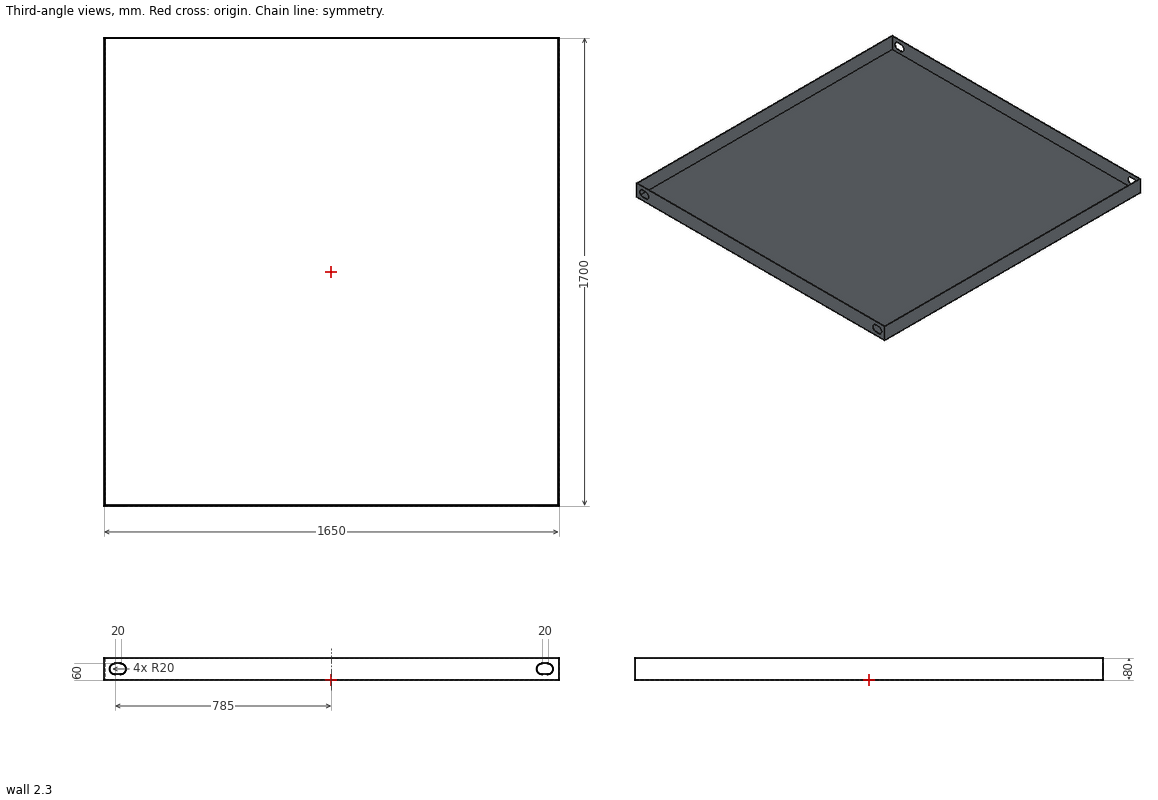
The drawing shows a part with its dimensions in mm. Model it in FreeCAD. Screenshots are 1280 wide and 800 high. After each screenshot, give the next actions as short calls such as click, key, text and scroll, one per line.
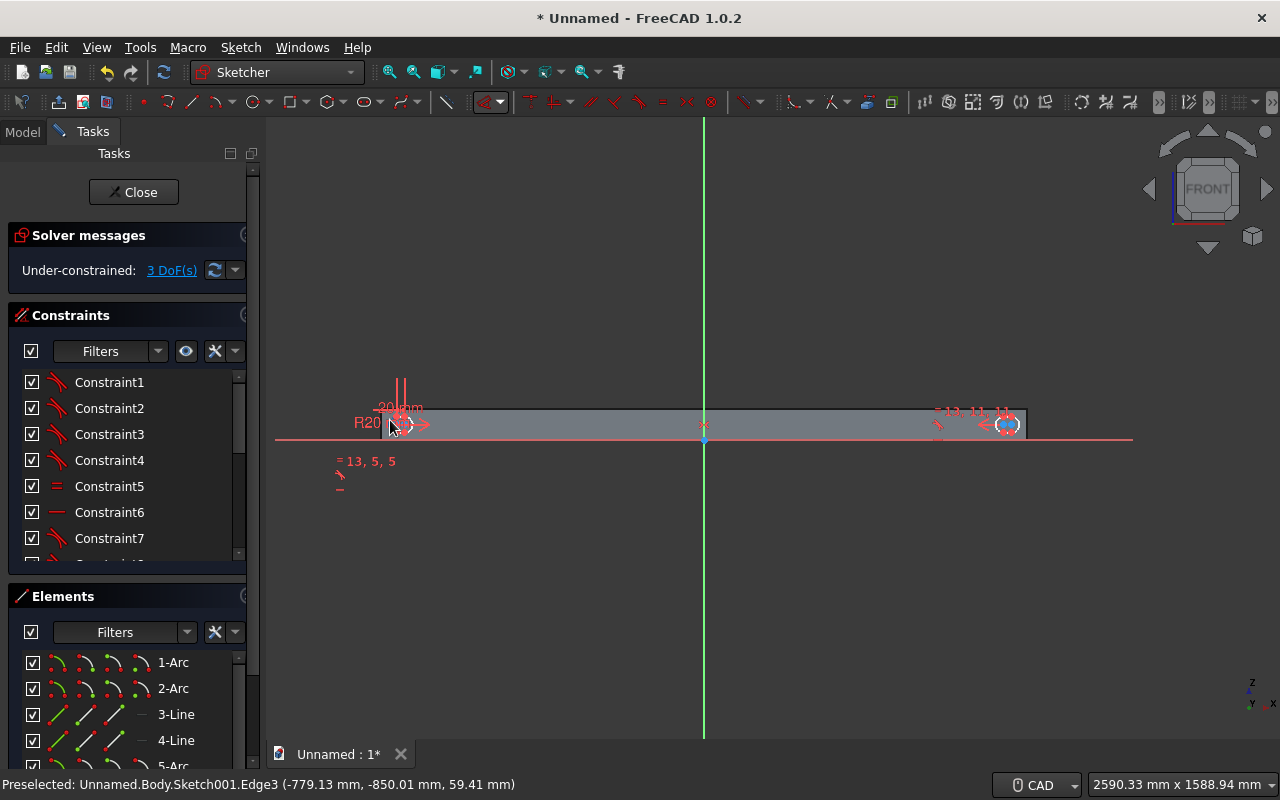
scroll(1006, 417, up, 9)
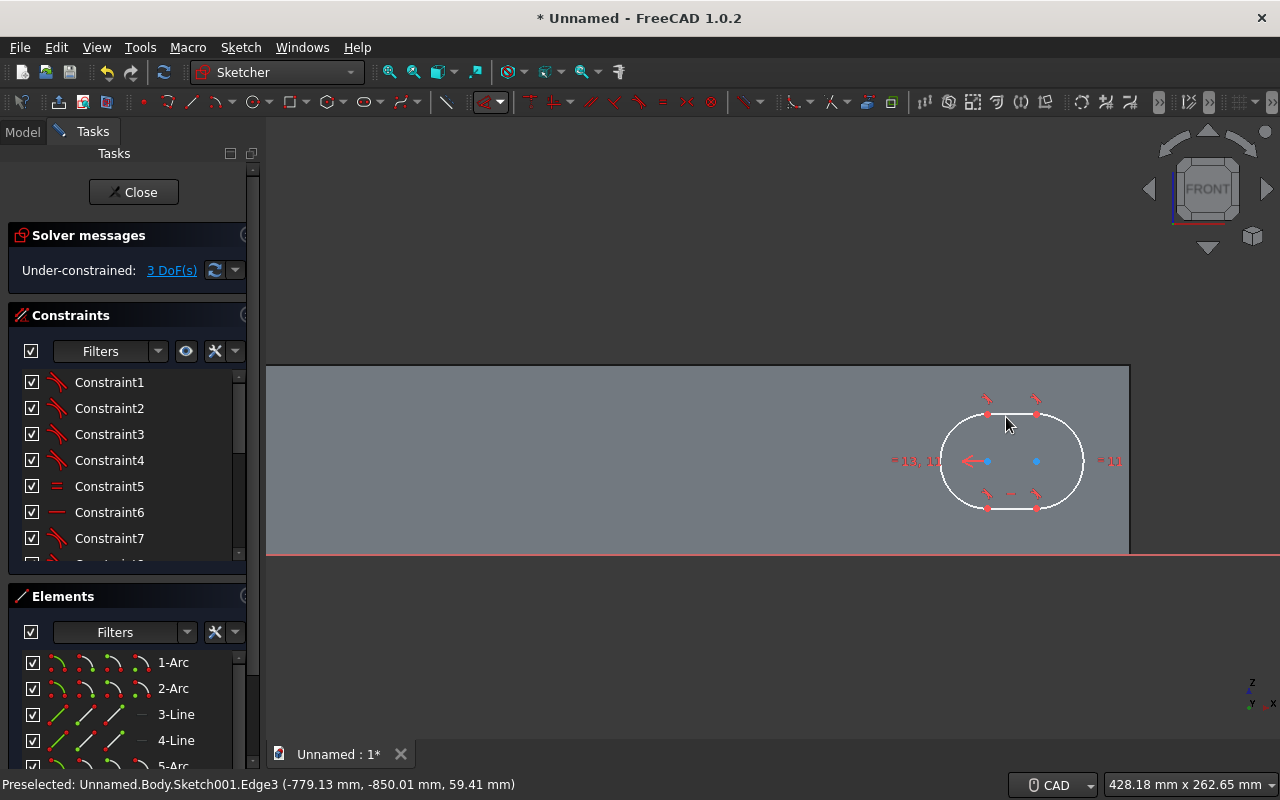
click(1002, 414)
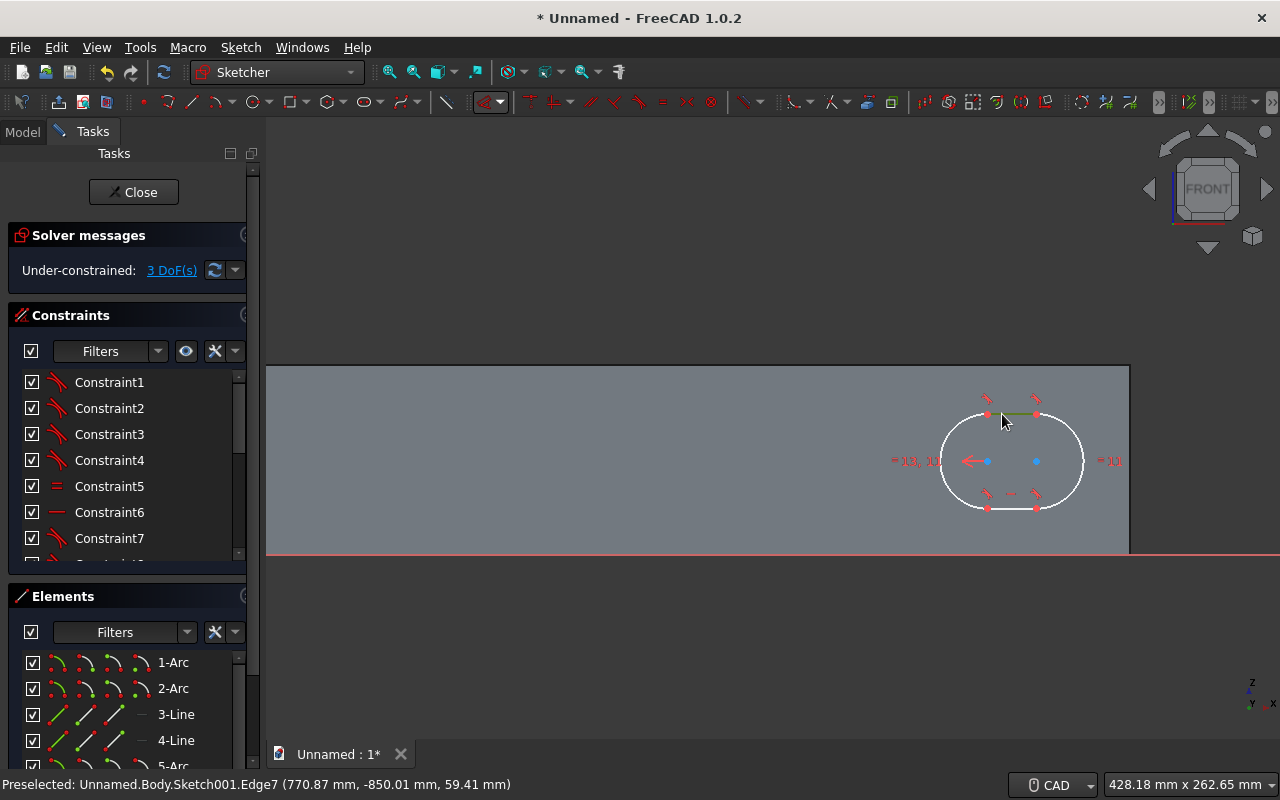
key(l)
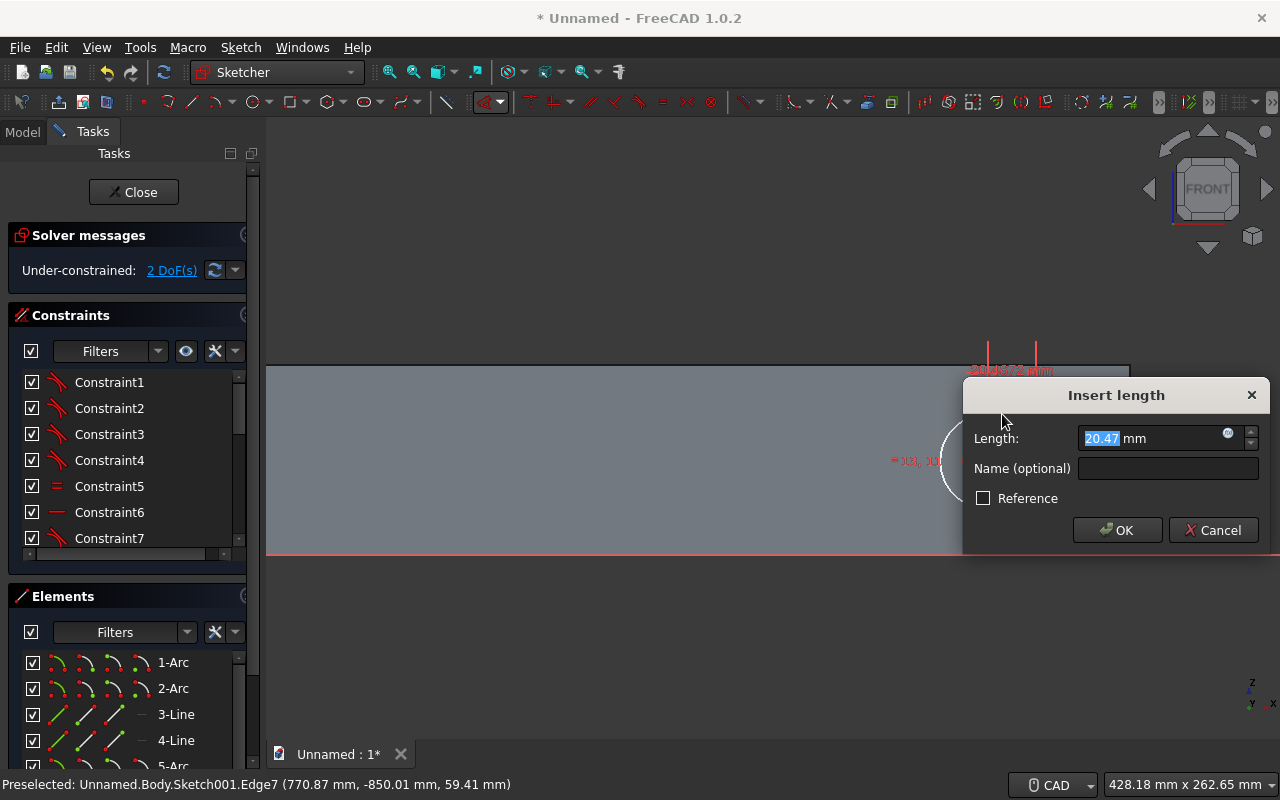
text(20)
key(Return)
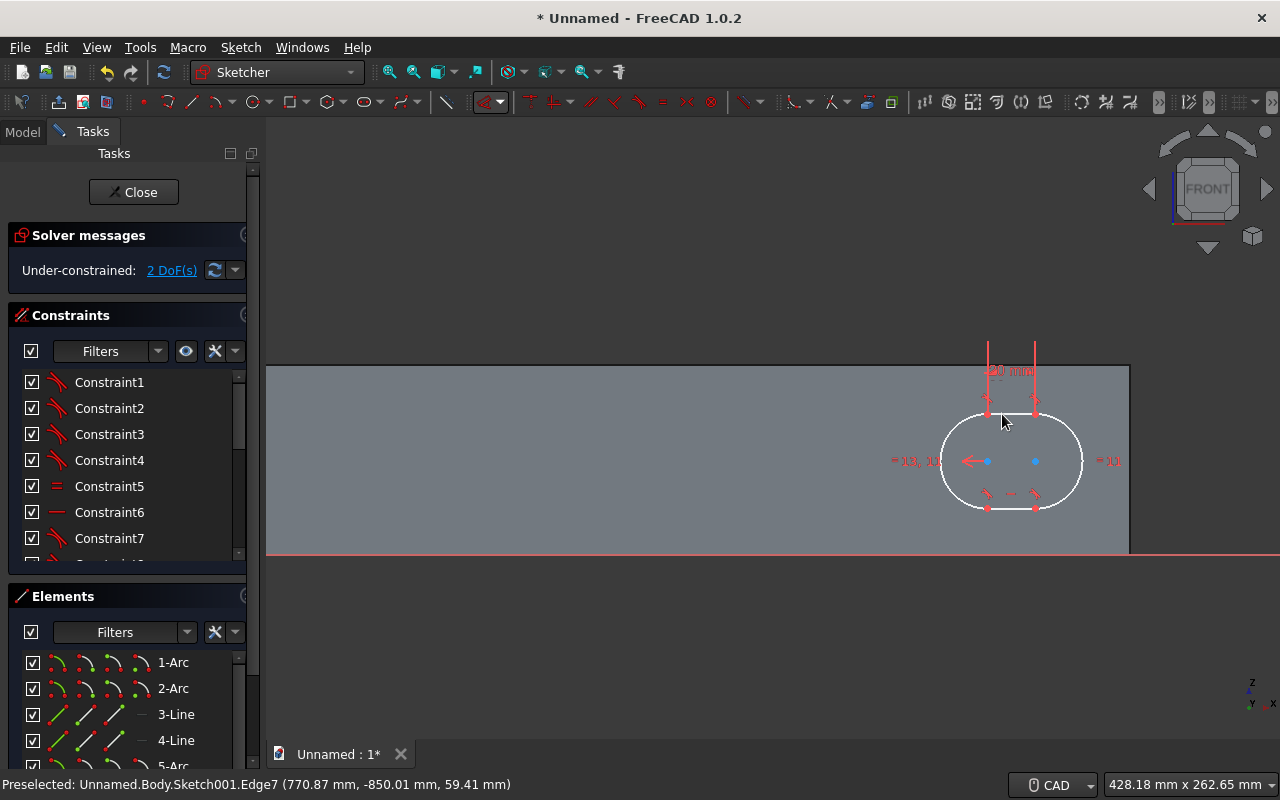
scroll(1007, 417, down, 9)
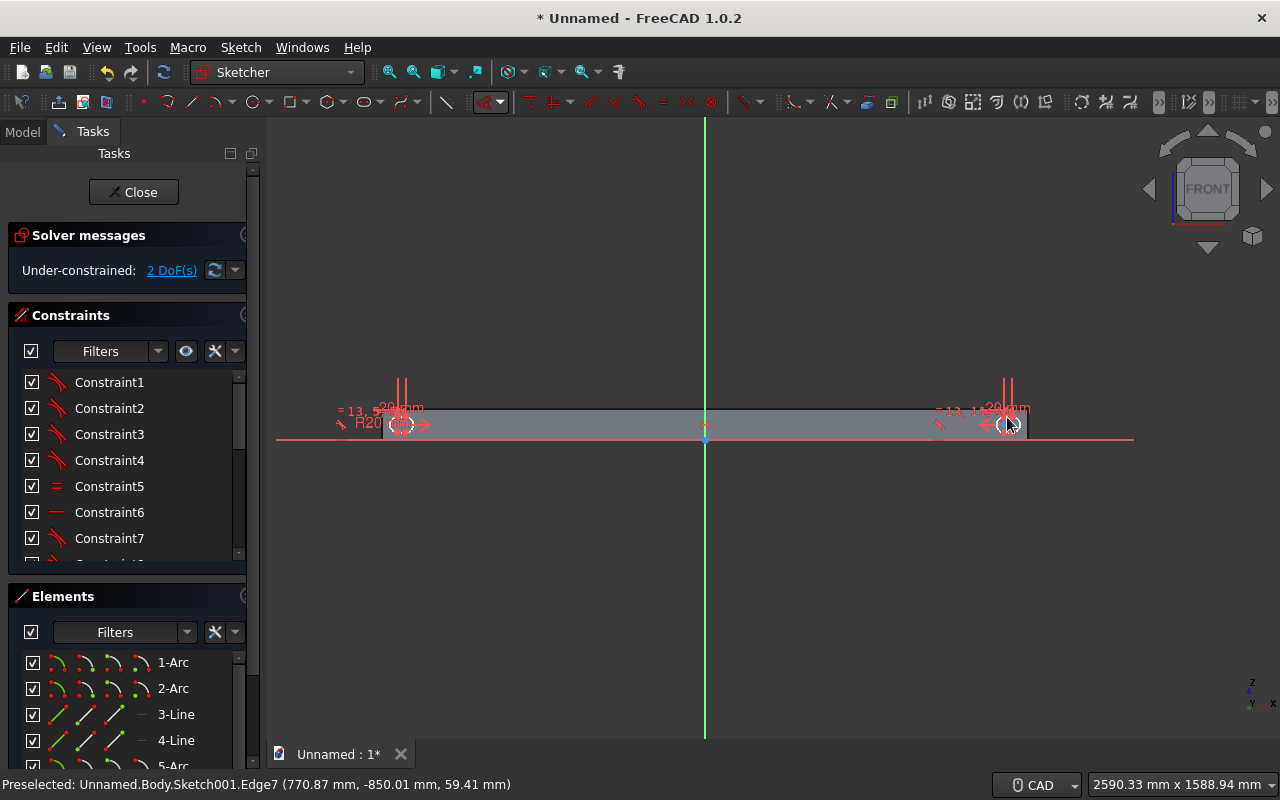
scroll(398, 417, up, 3)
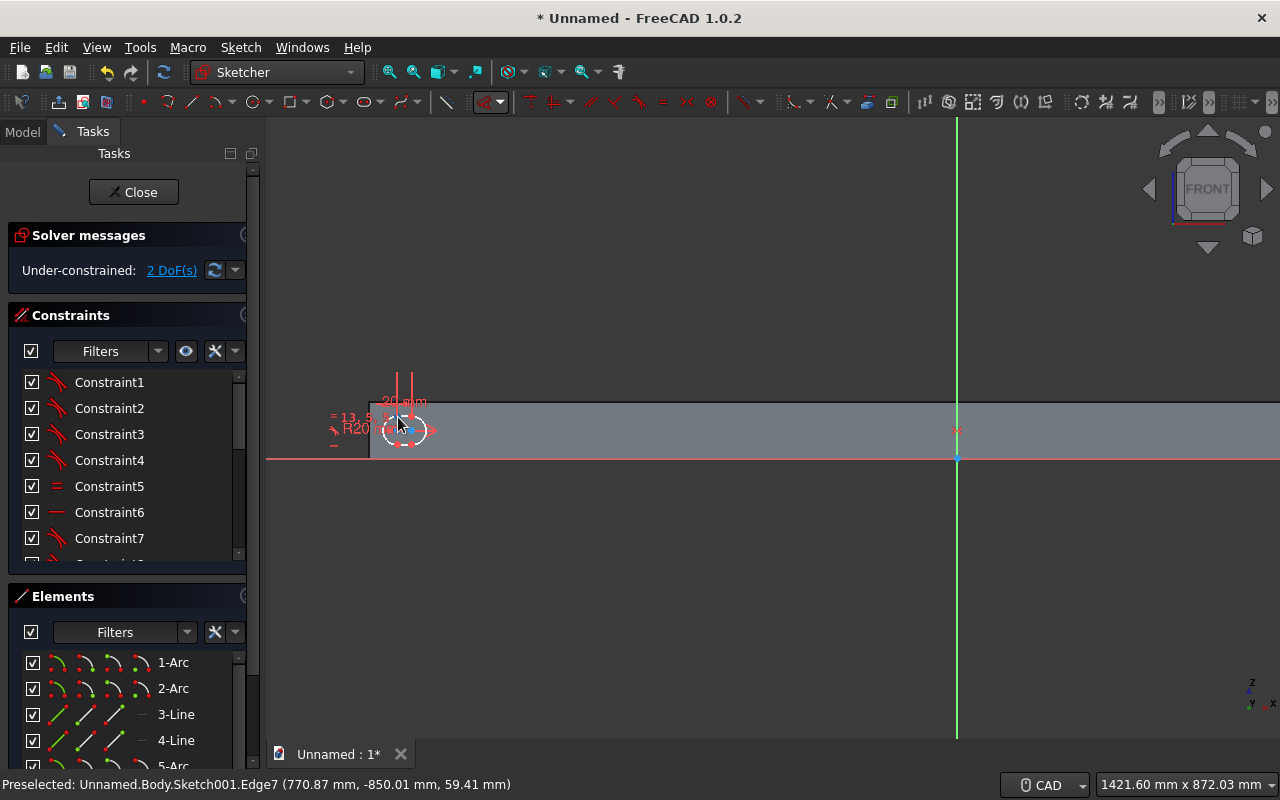
click(397, 416)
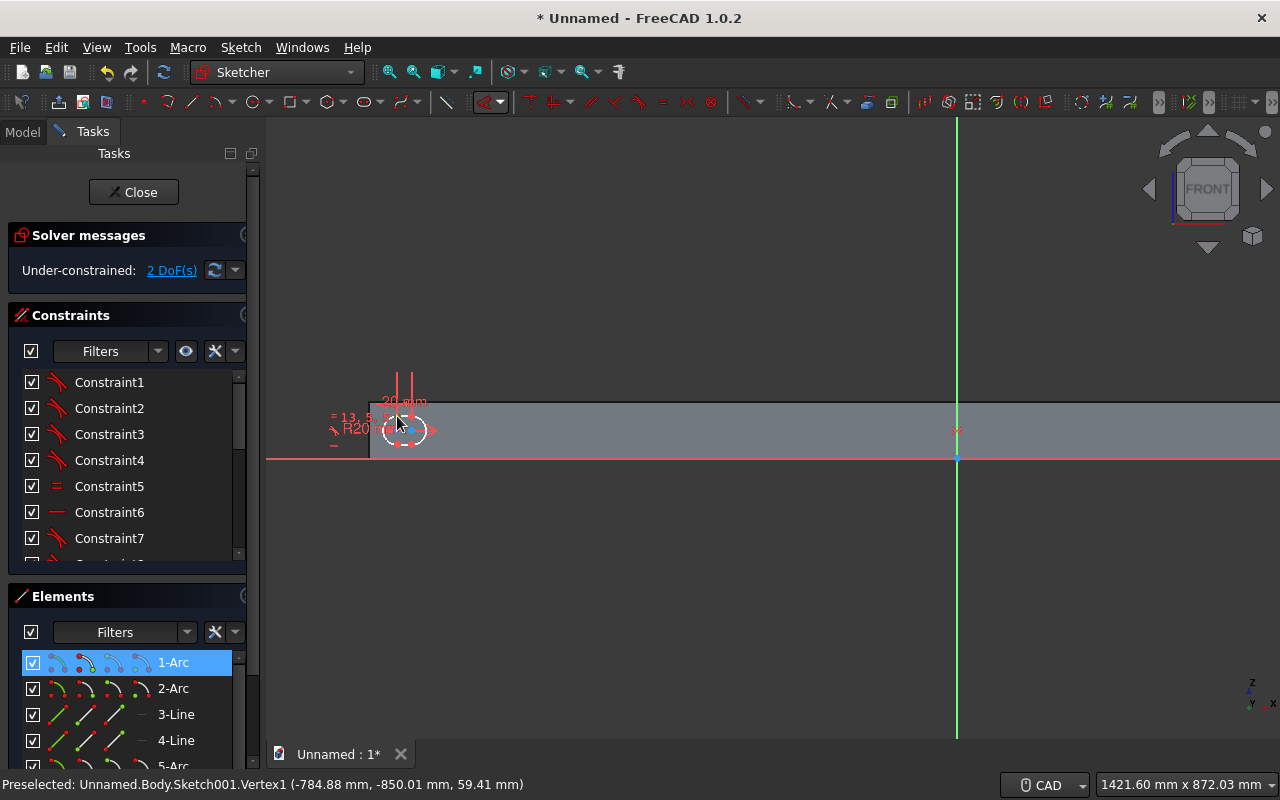
key(i)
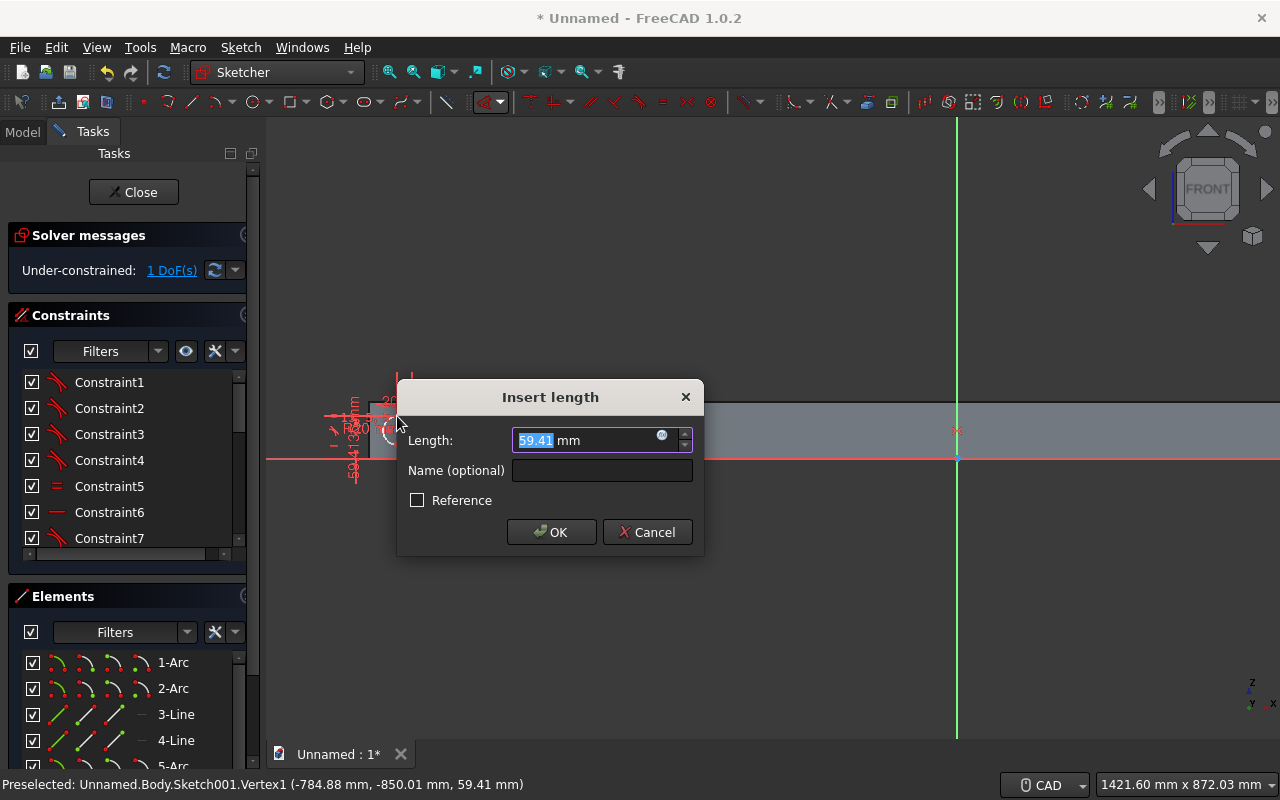
text(60)
key(Return)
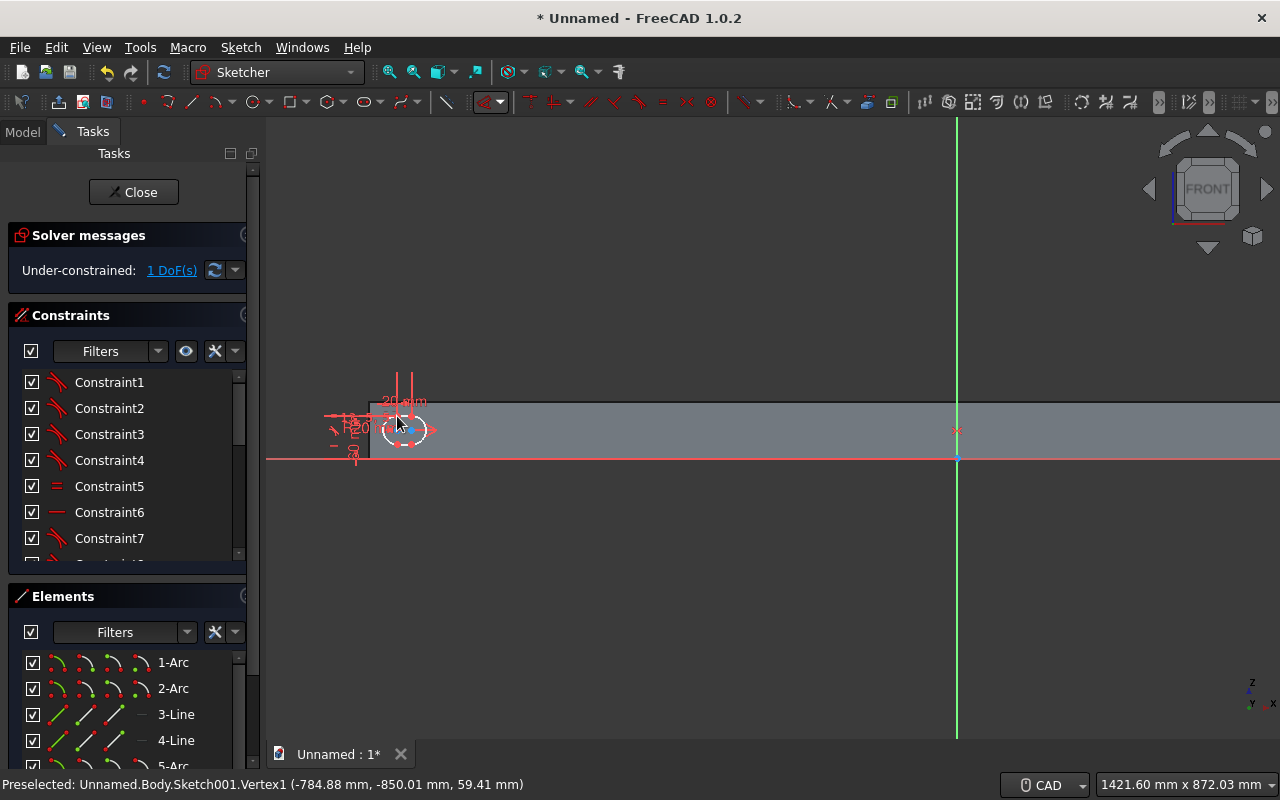
click(397, 416)